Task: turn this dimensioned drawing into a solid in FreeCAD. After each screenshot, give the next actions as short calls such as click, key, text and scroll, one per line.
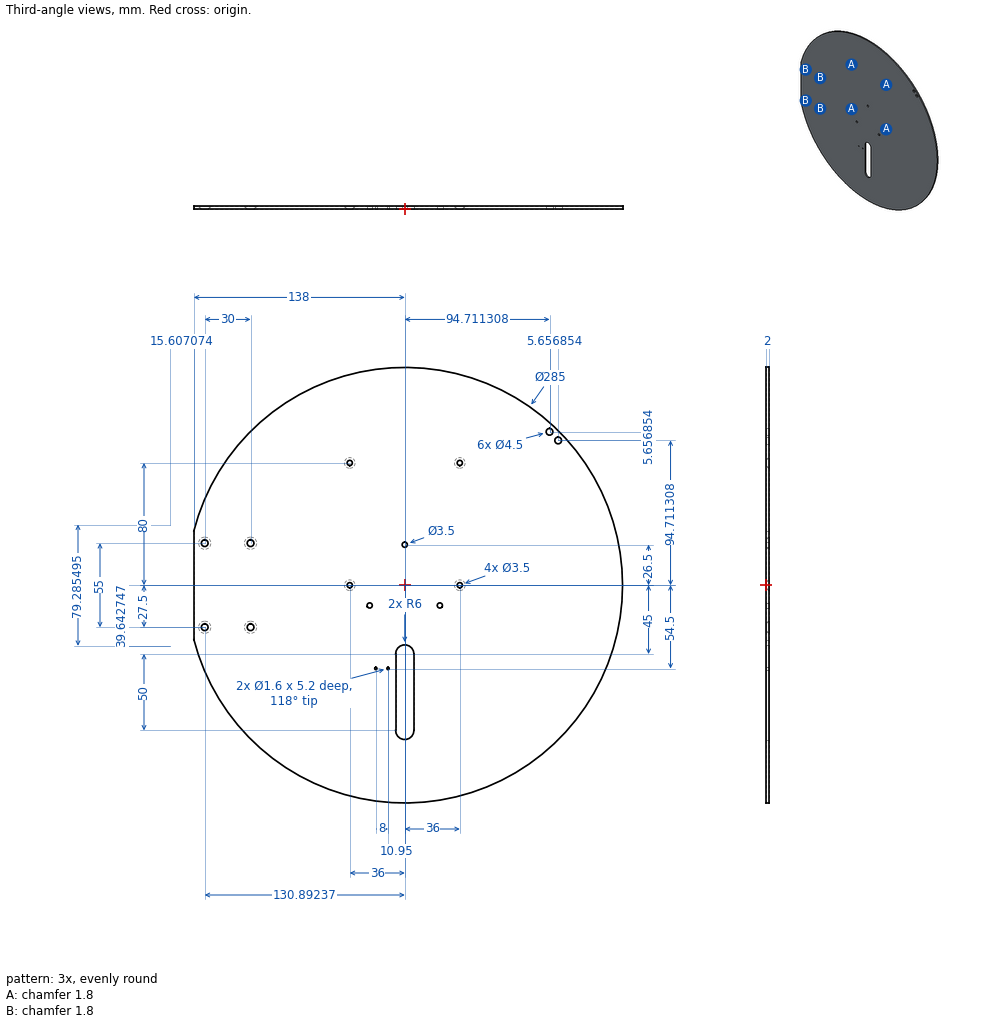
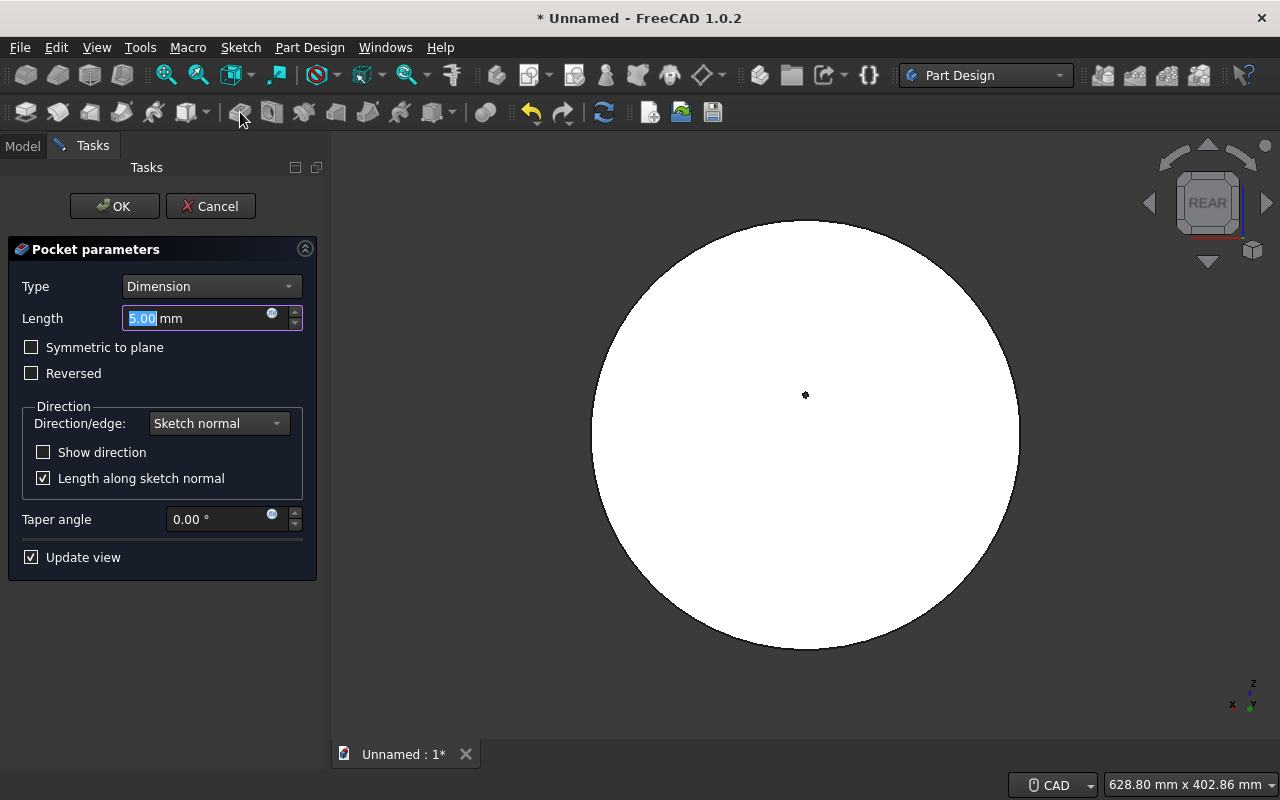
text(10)
key(Tab)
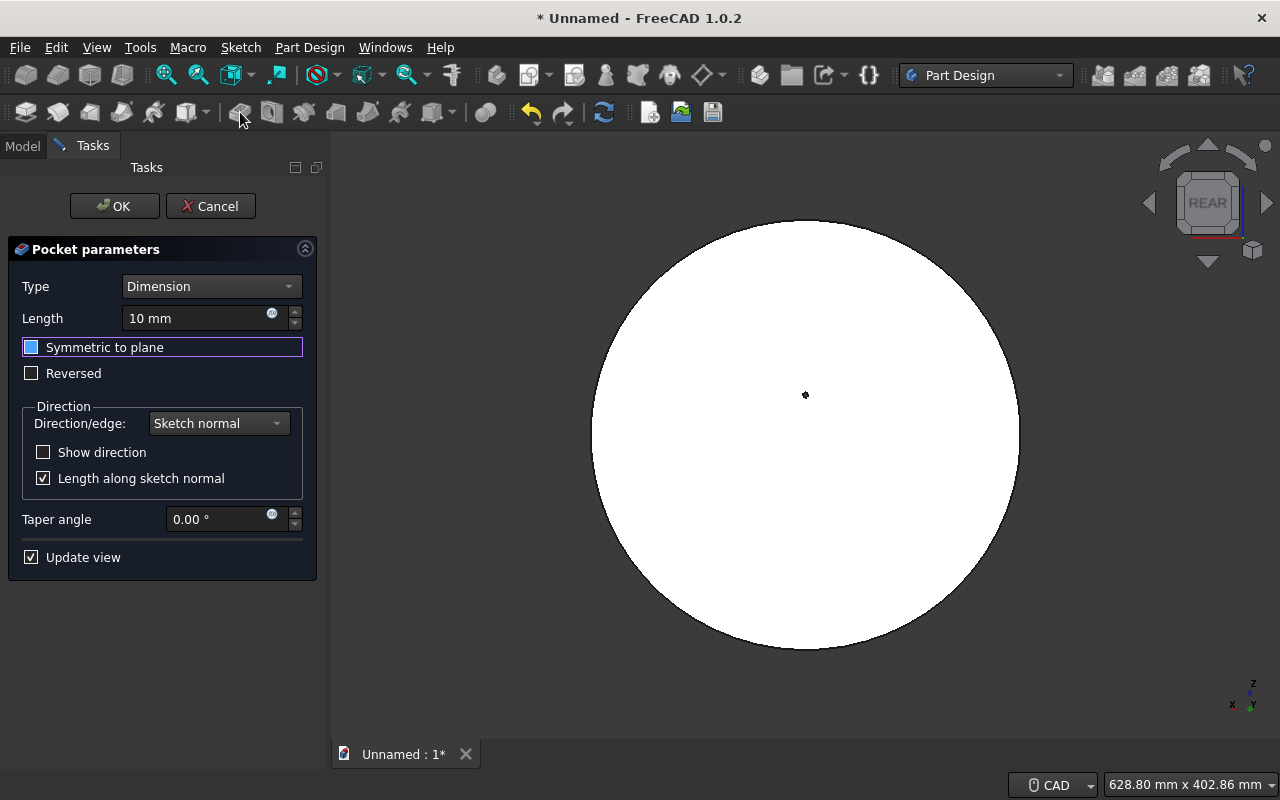
click(115, 206)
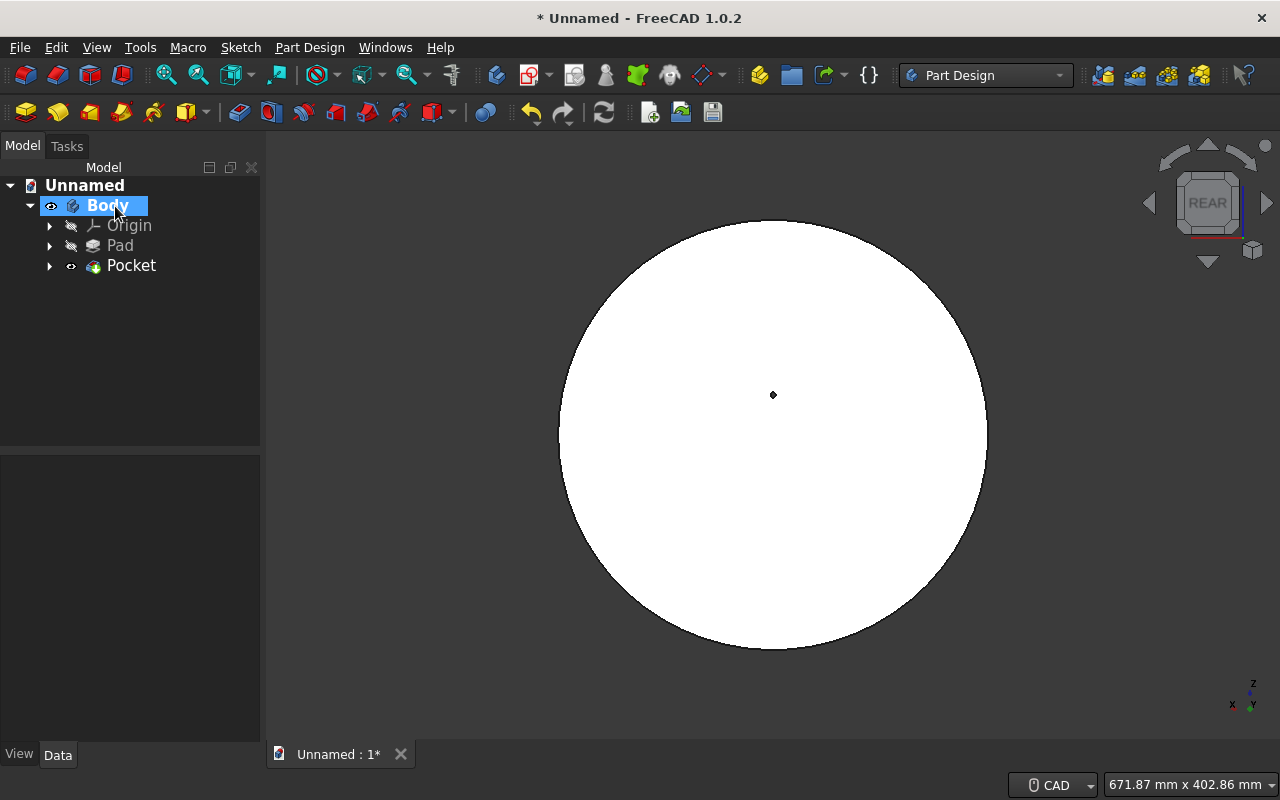
click(116, 266)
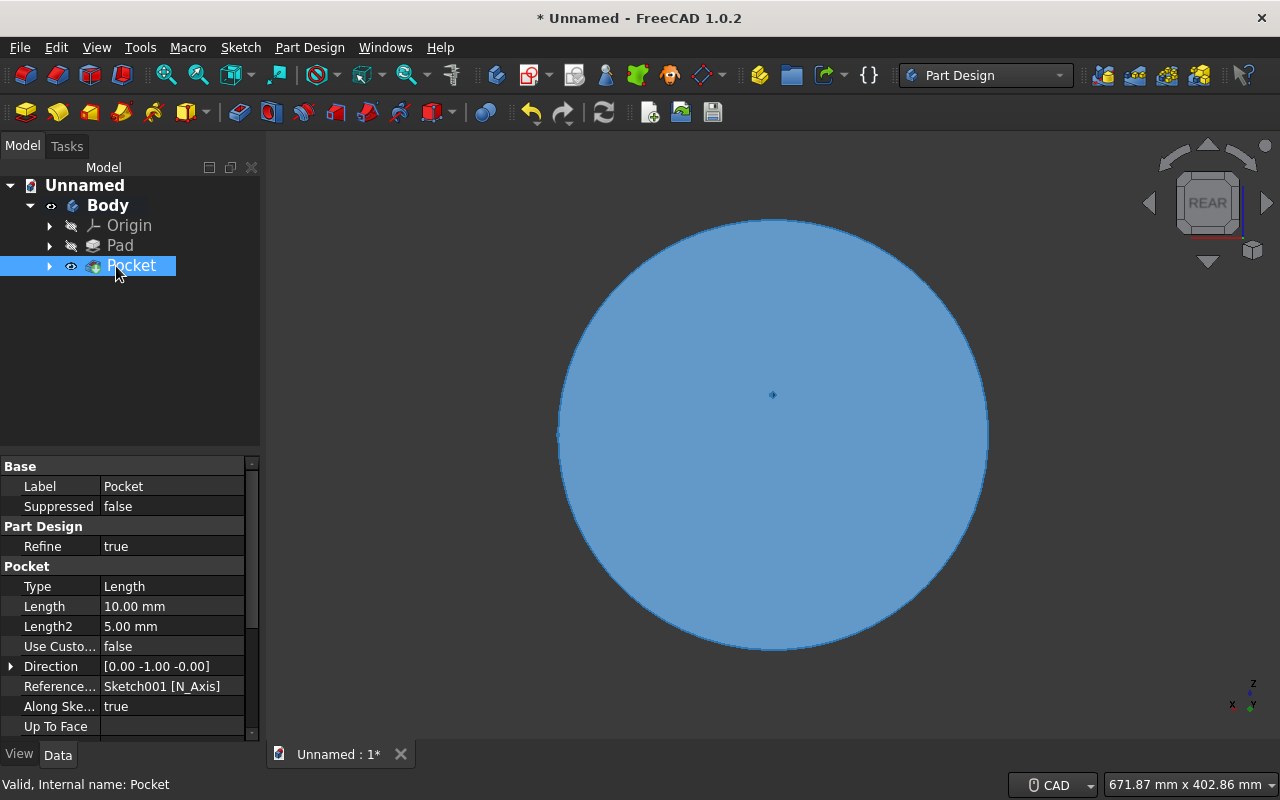
click(1168, 76)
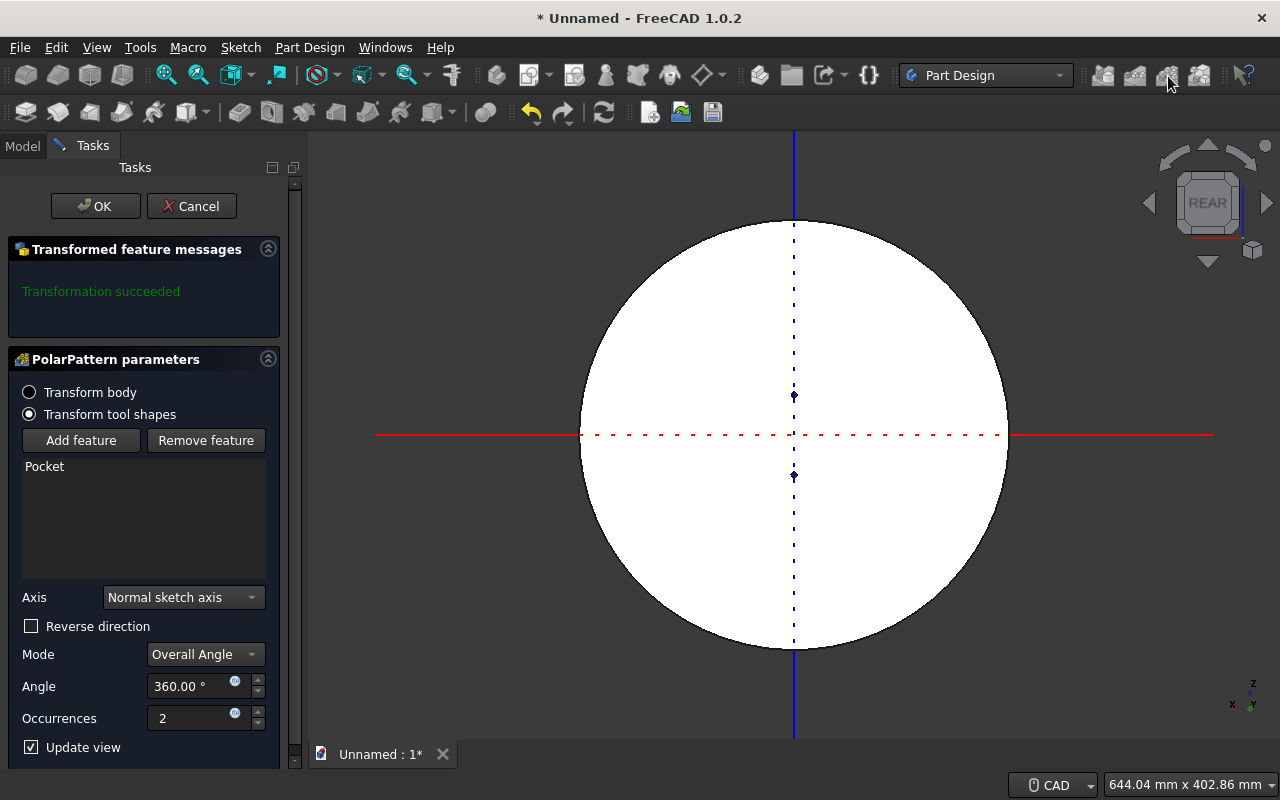
click(184, 598)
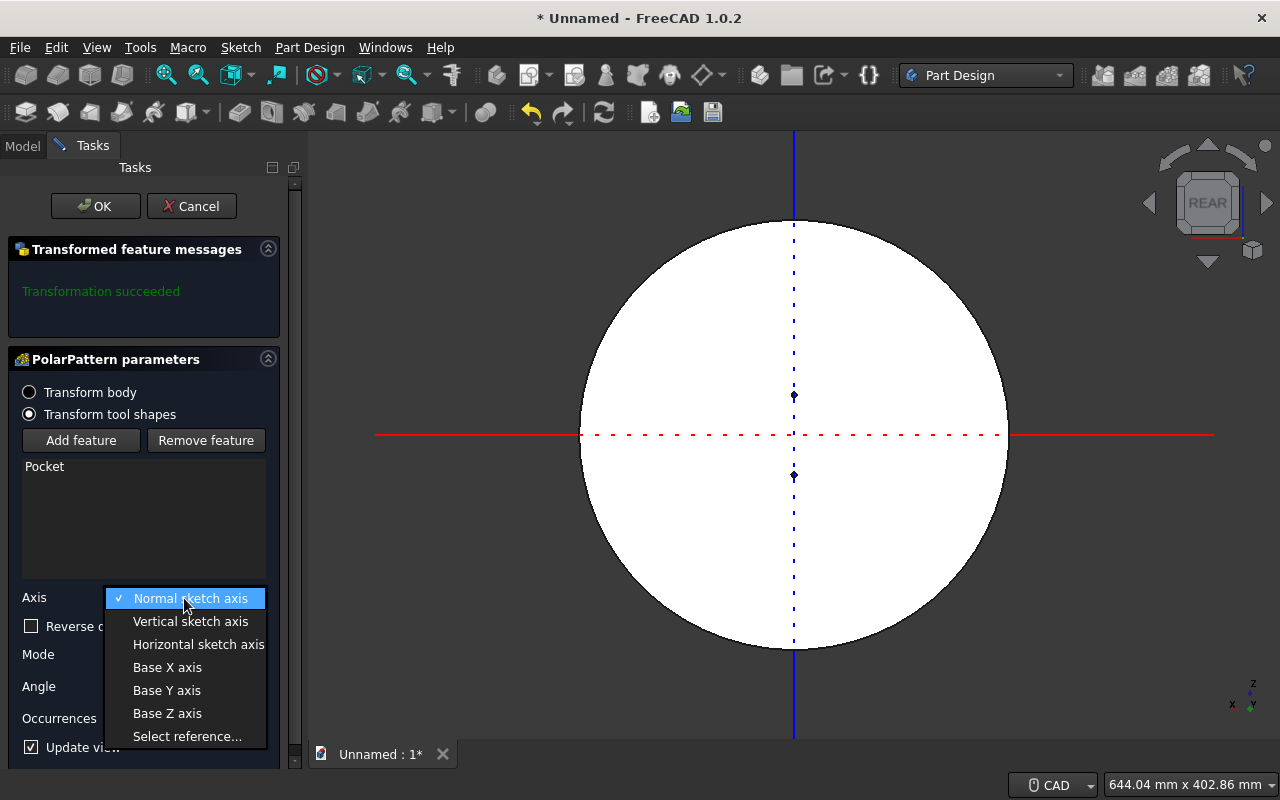
click(184, 690)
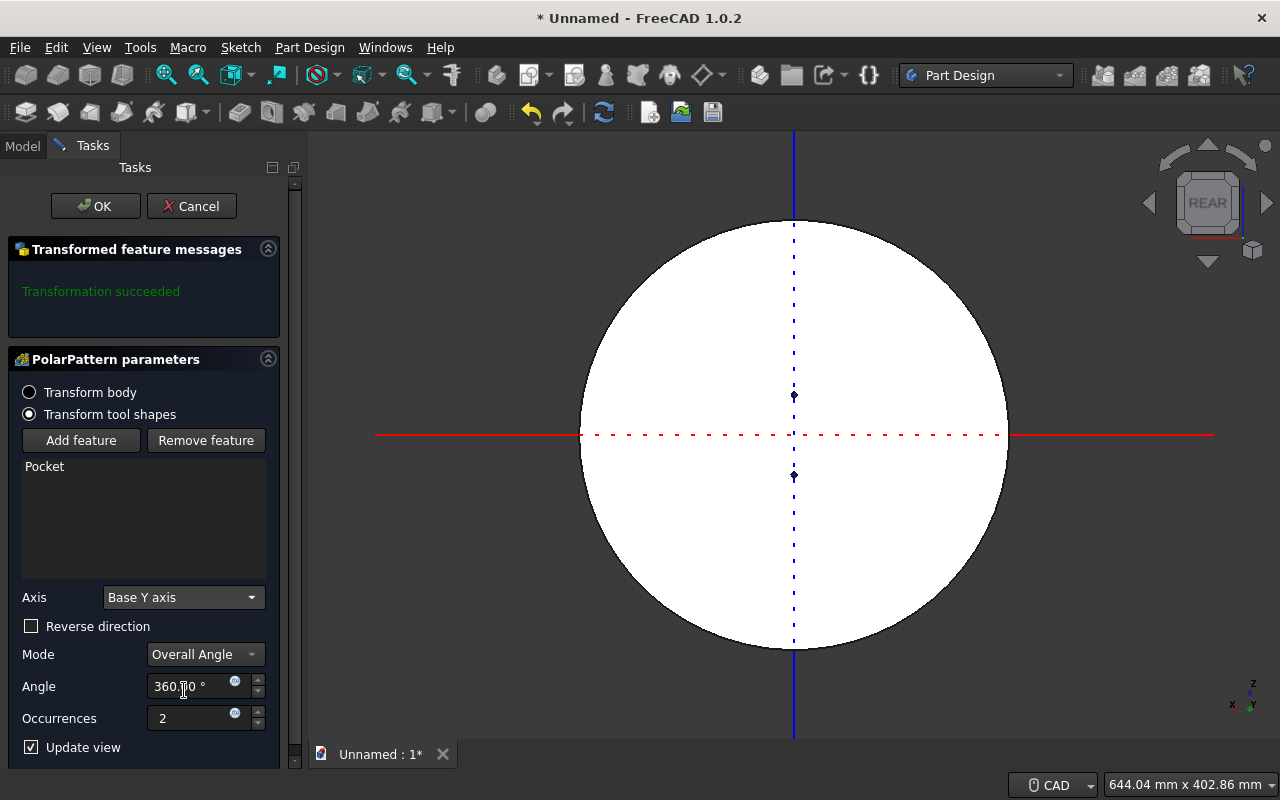
triple_click(198, 718)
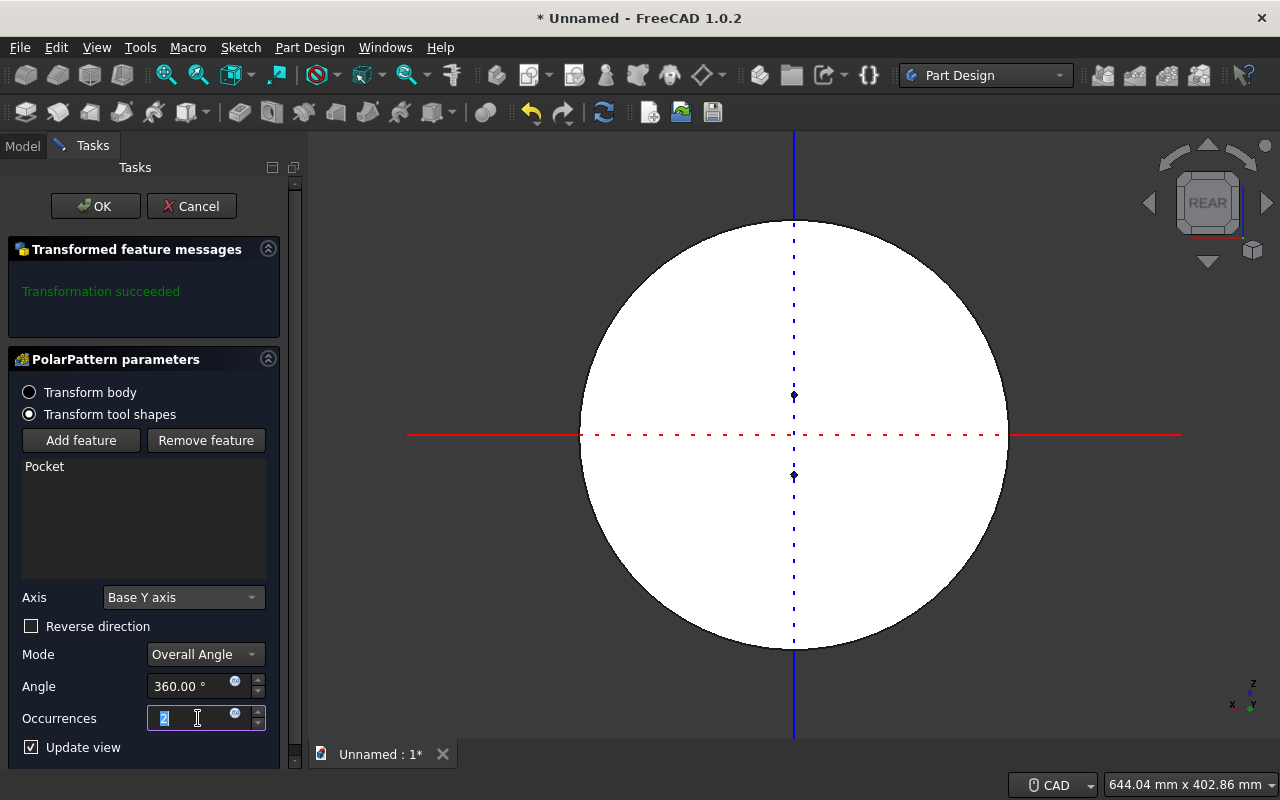
text(3)
key(Tab)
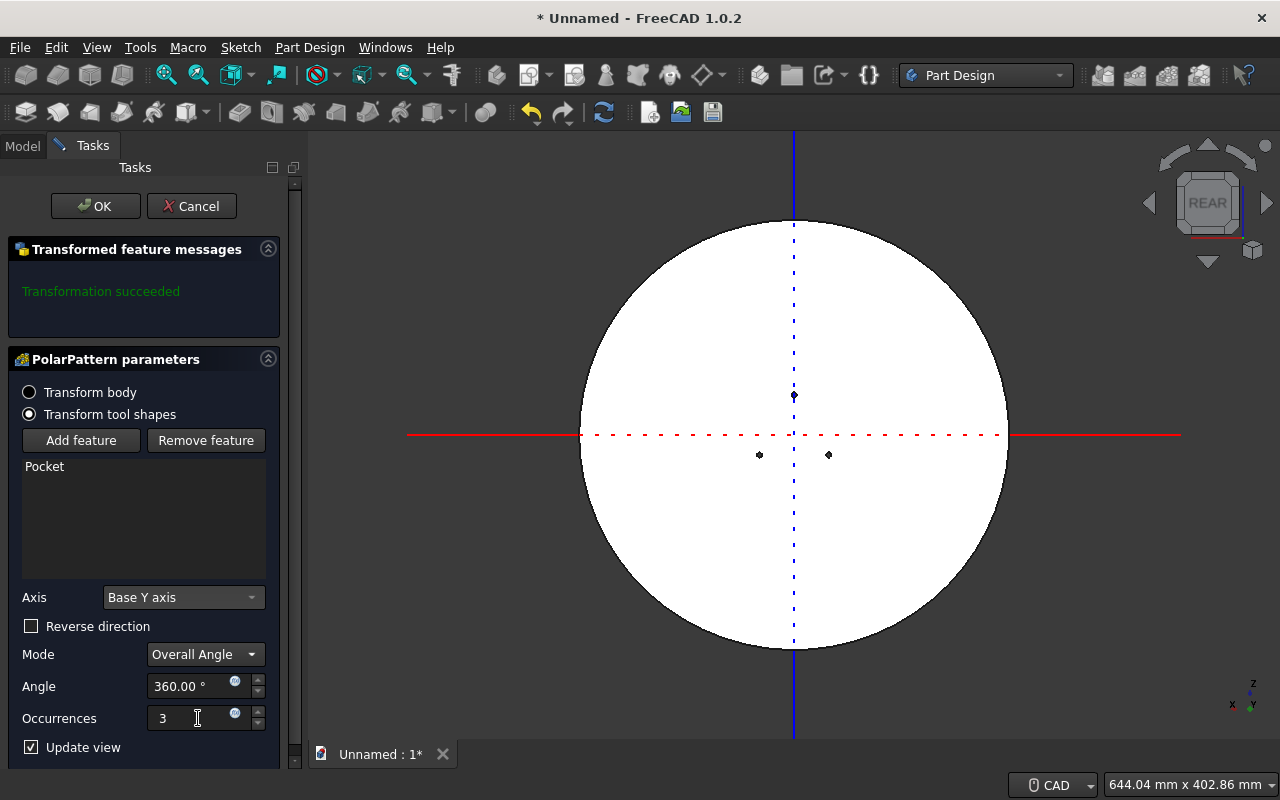
click(96, 206)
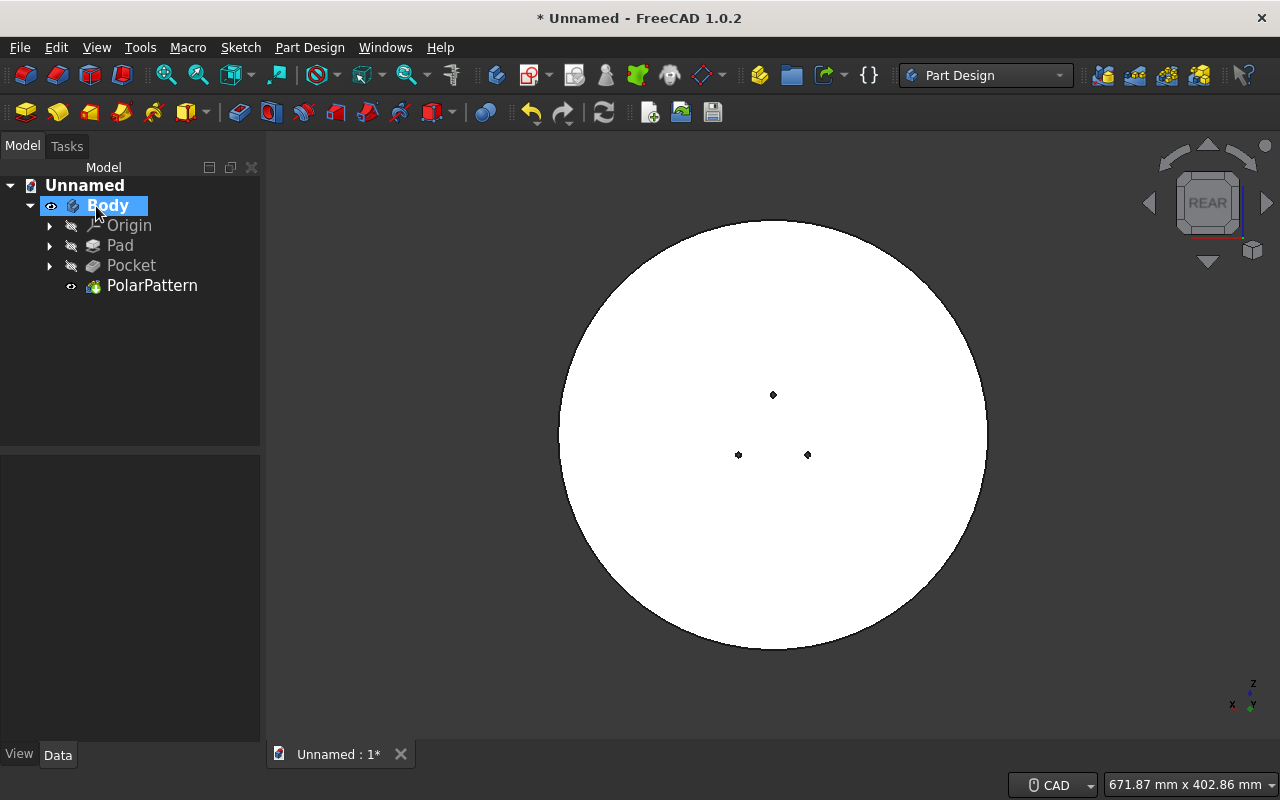
click(773, 557)